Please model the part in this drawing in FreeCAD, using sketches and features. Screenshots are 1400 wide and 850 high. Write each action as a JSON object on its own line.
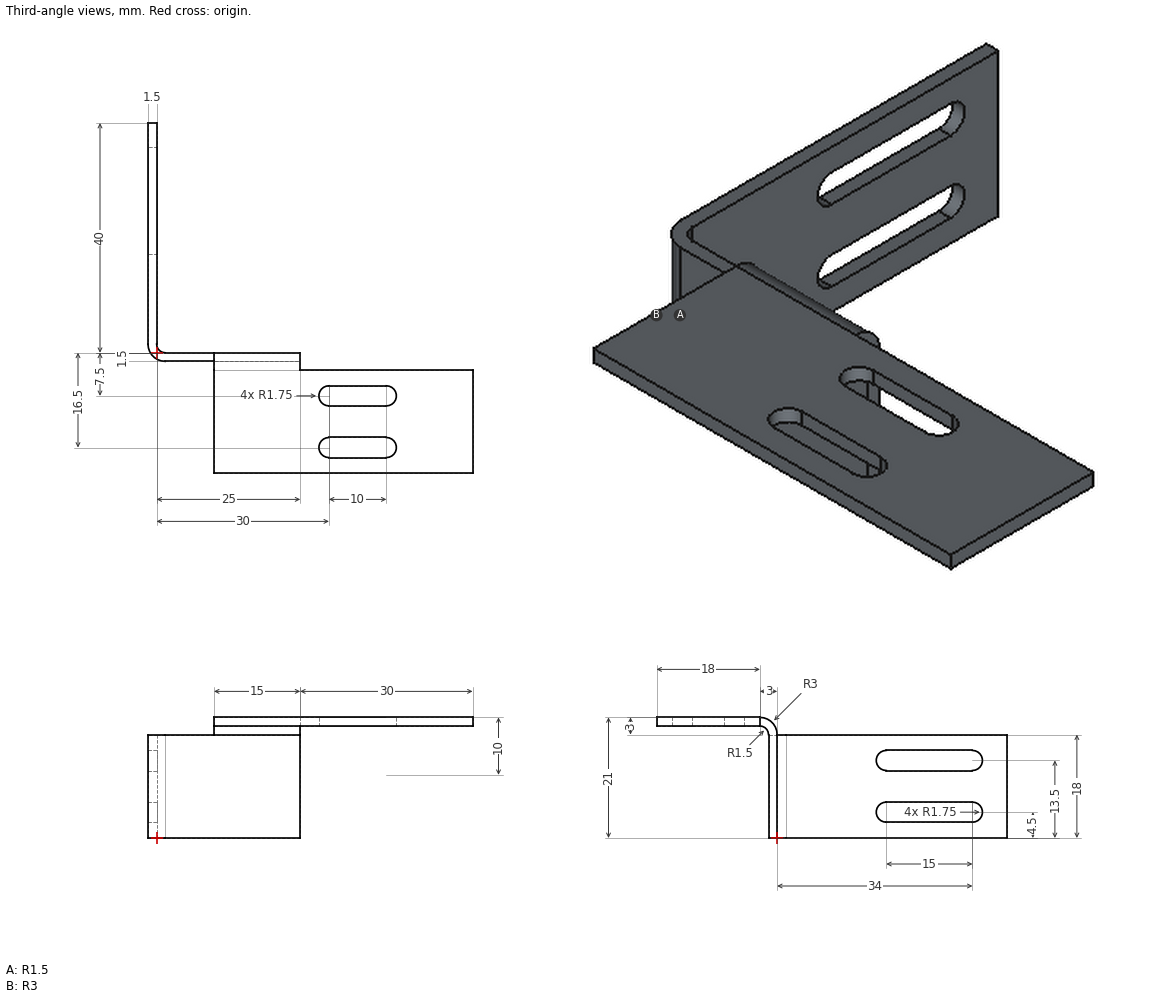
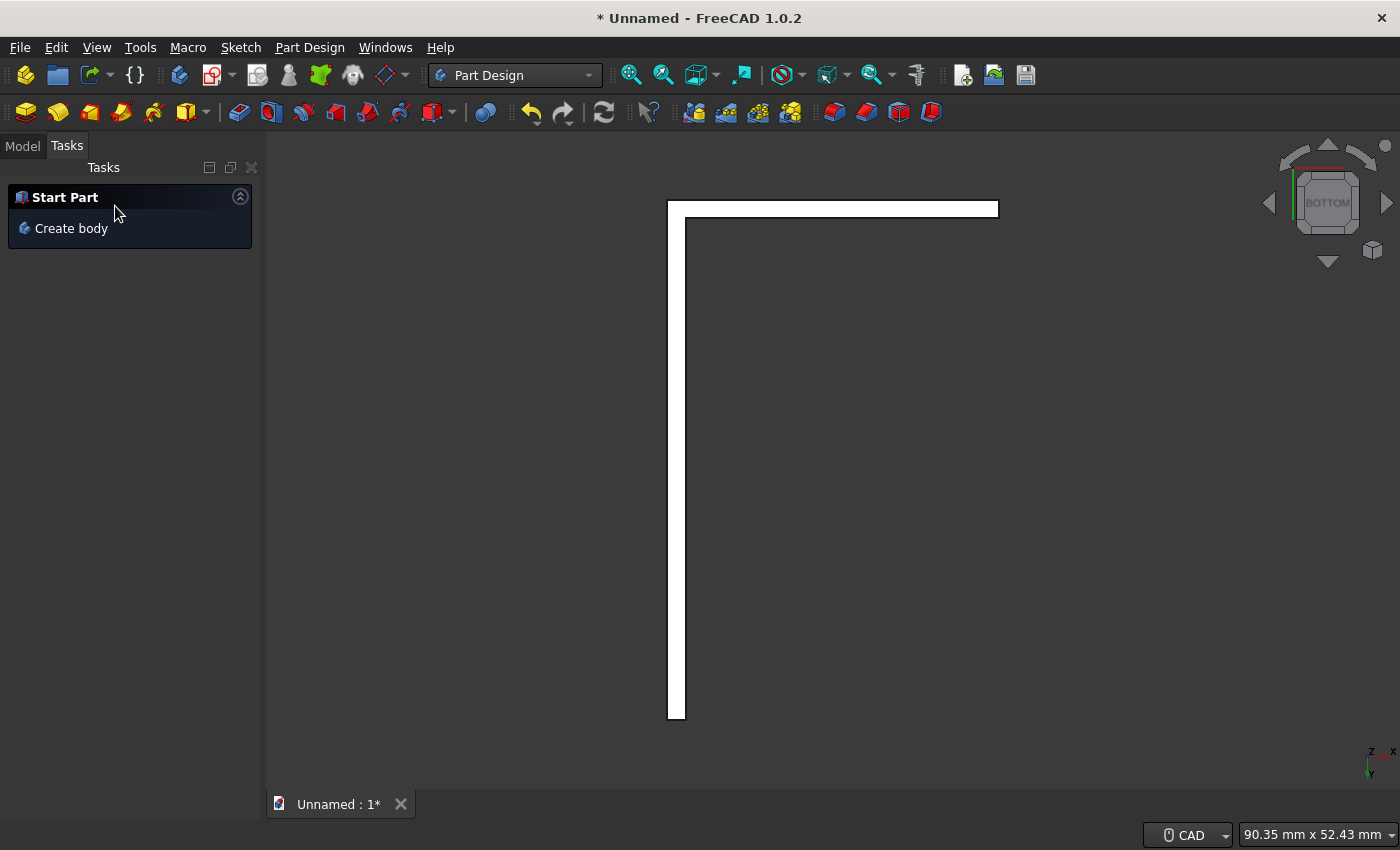
{"action": "key", "text": "4"}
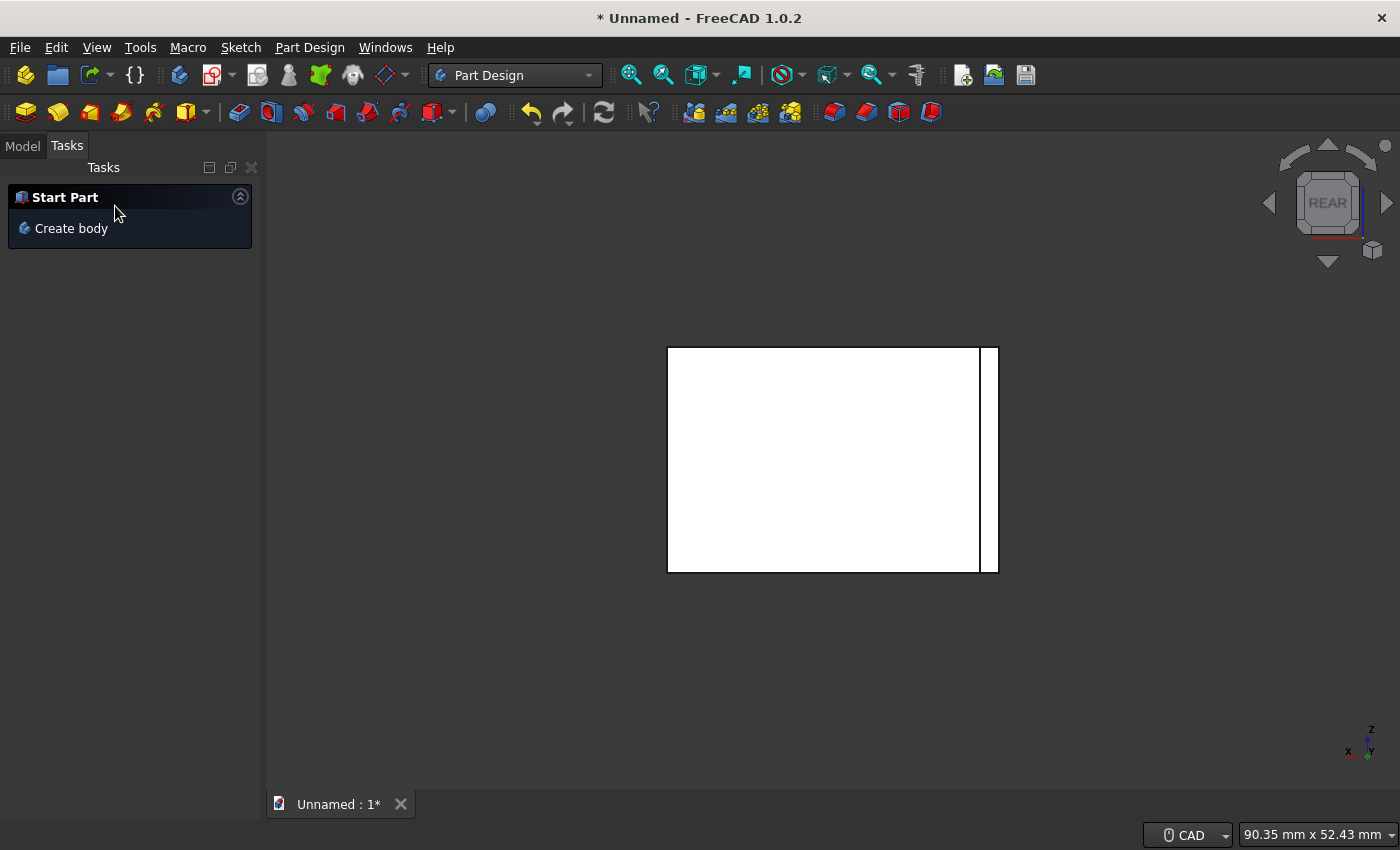
{"action": "key", "text": "v f"}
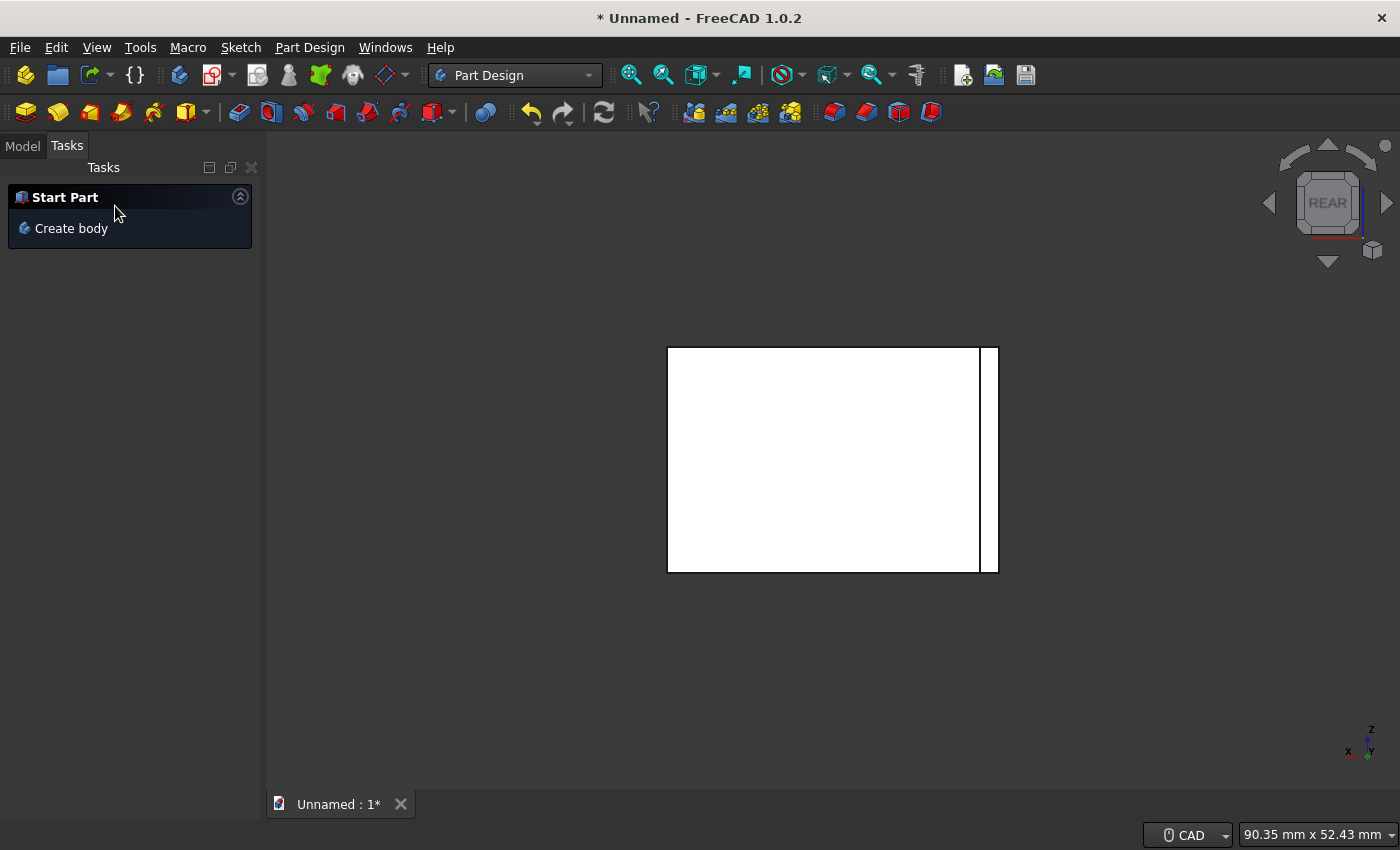
{"action": "key", "text": "6"}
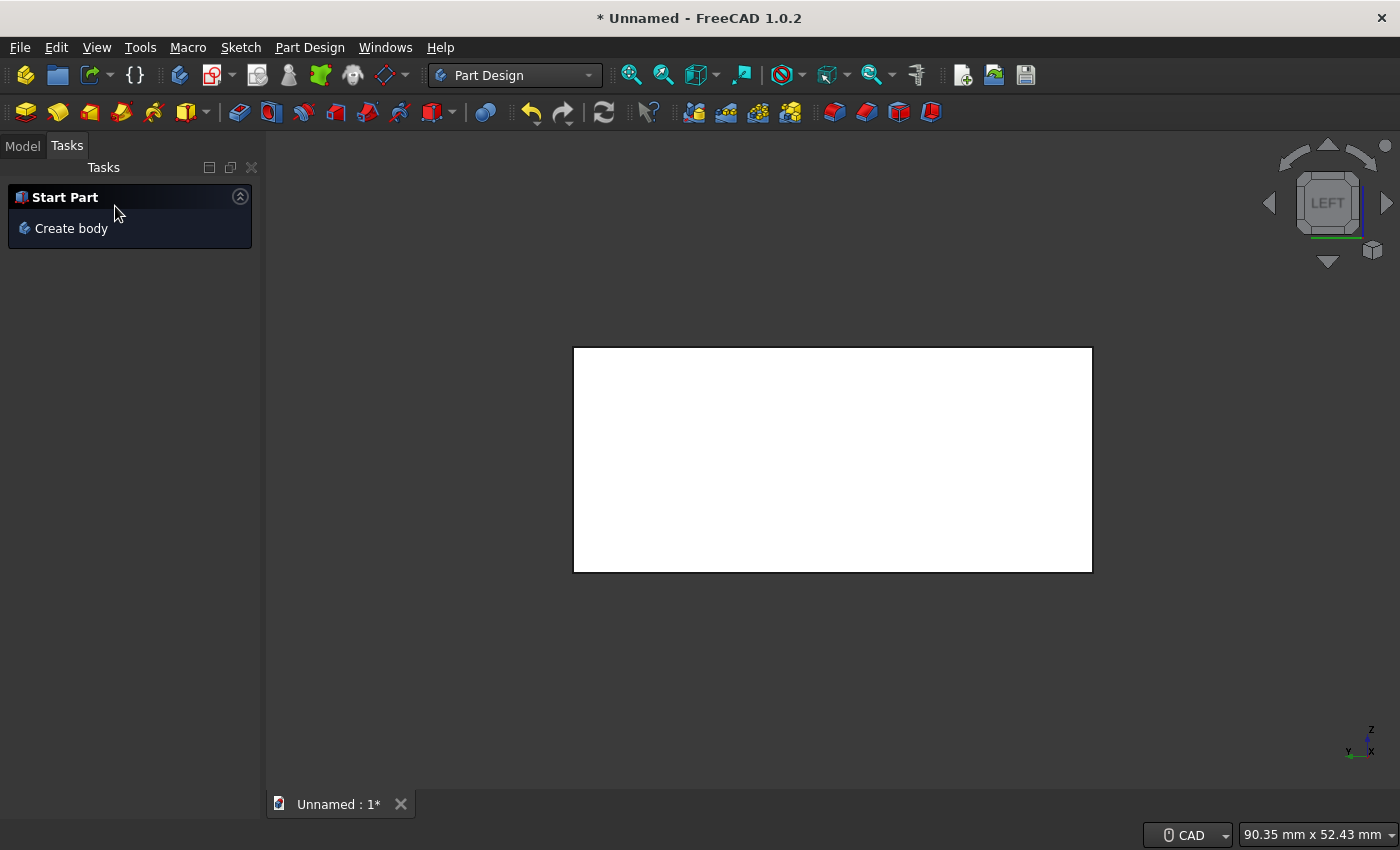
{"action": "key", "text": "v 3"}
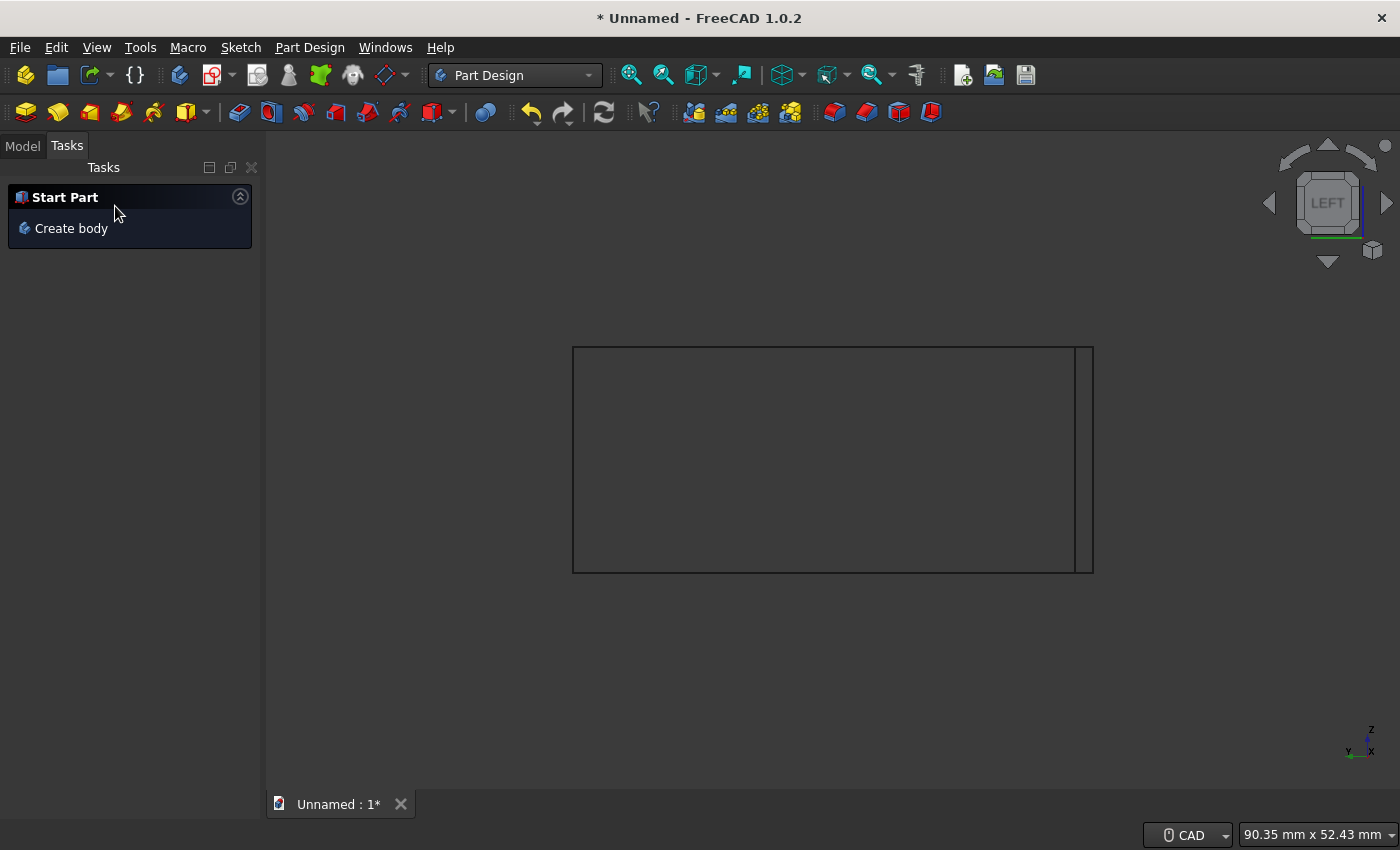
{"action": "key", "text": "0"}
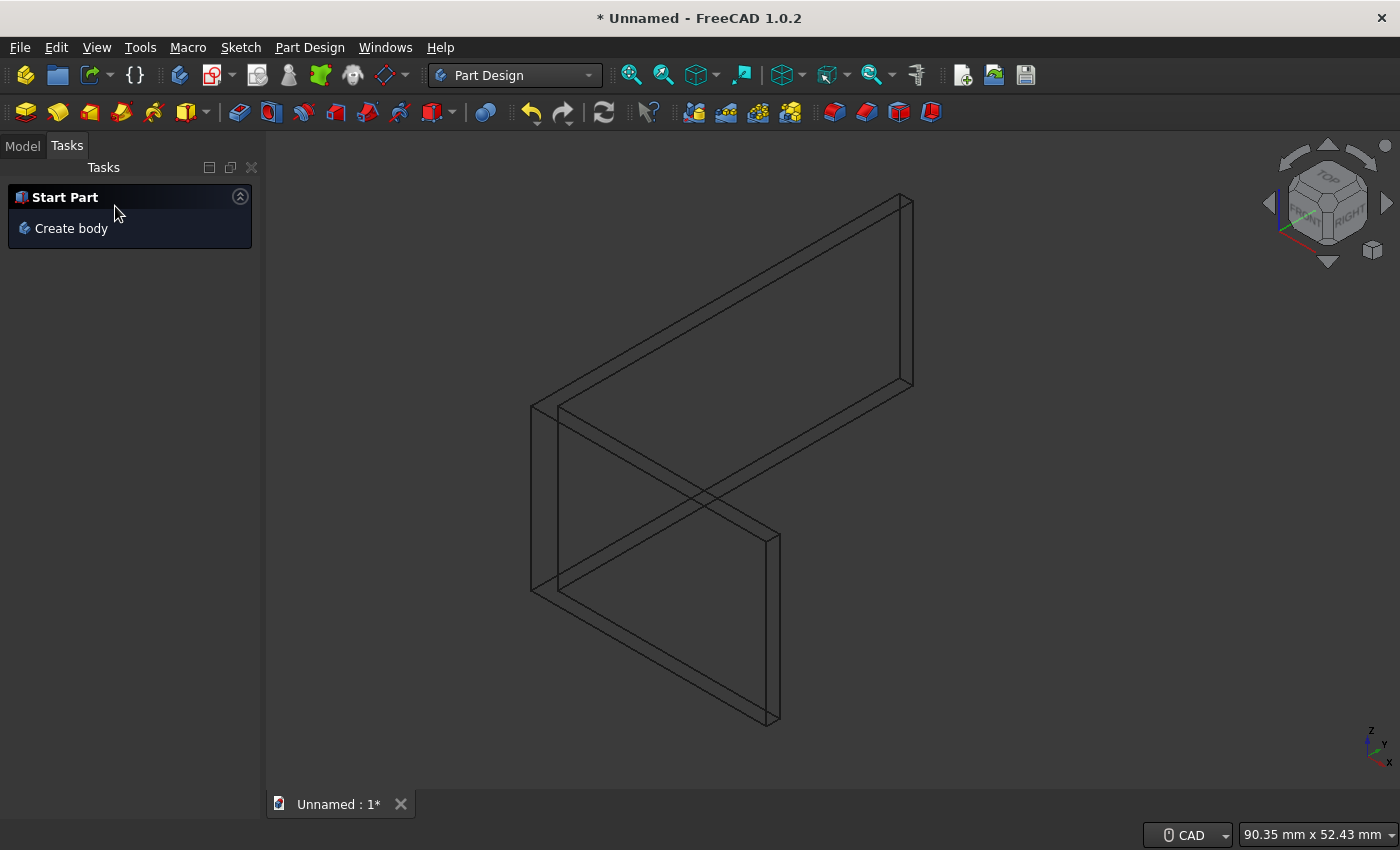
{"action": "left_click", "coordinate": [558, 497]}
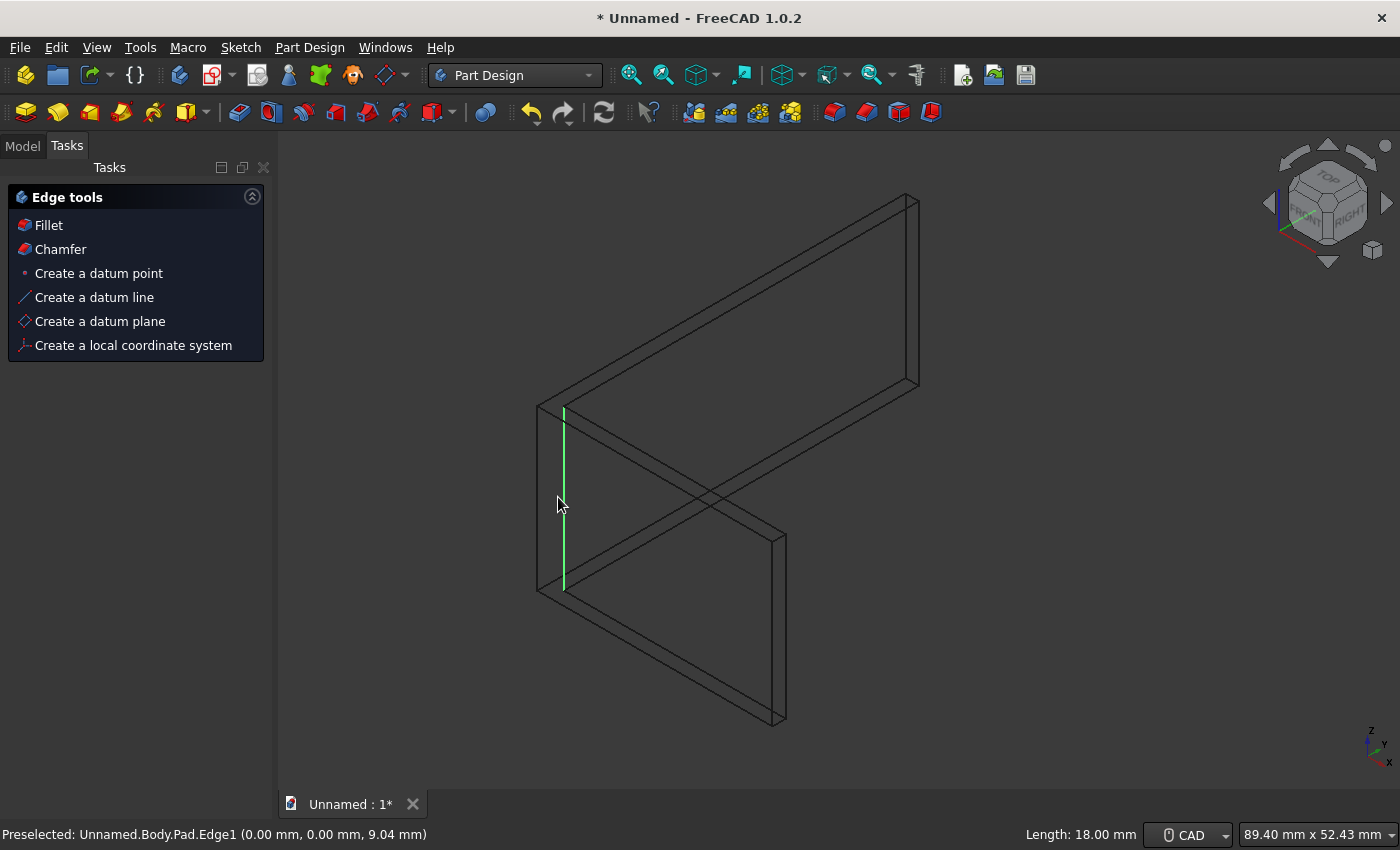
{"action": "key", "text": "v 1"}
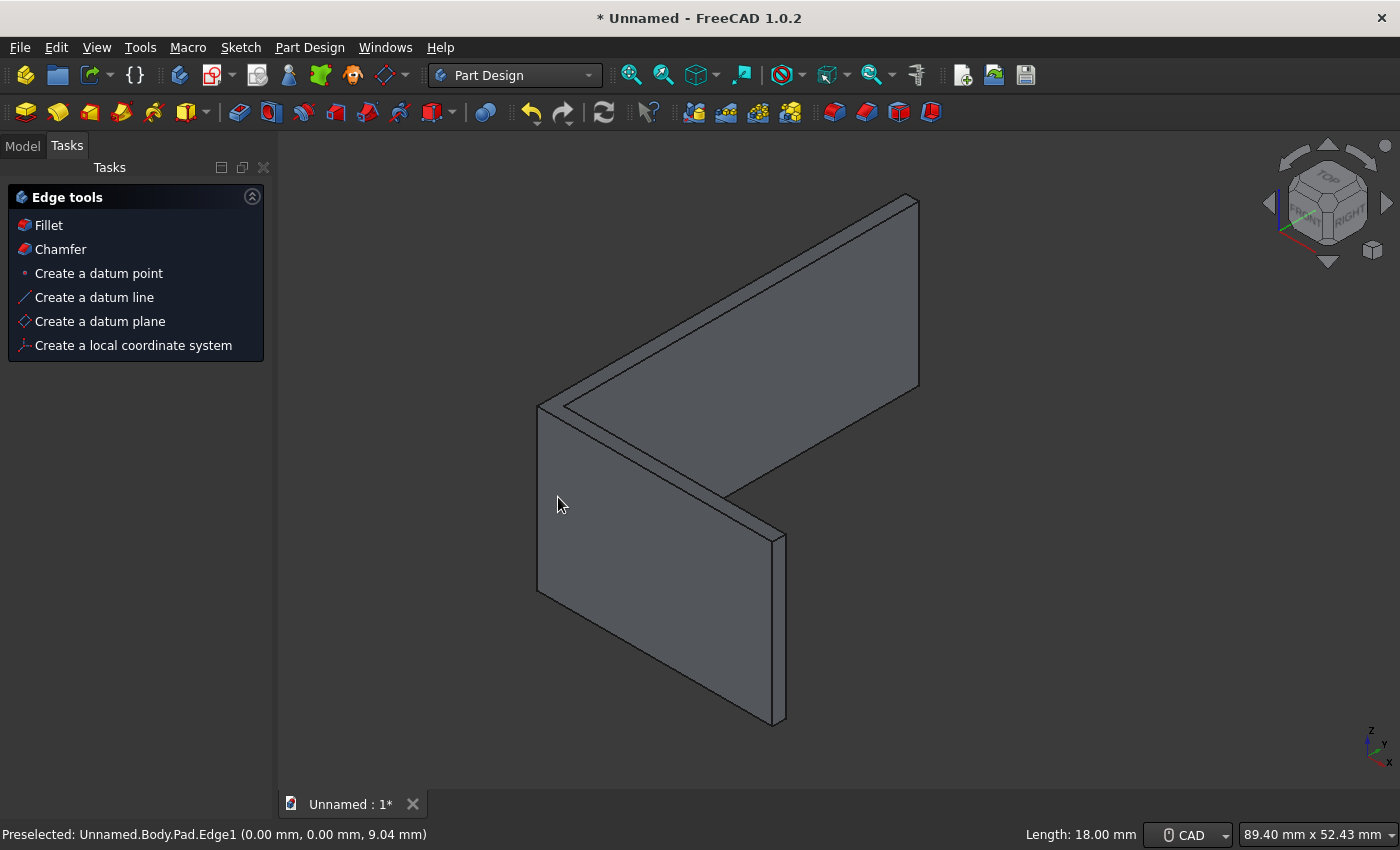
{"action": "left_click", "coordinate": [836, 112]}